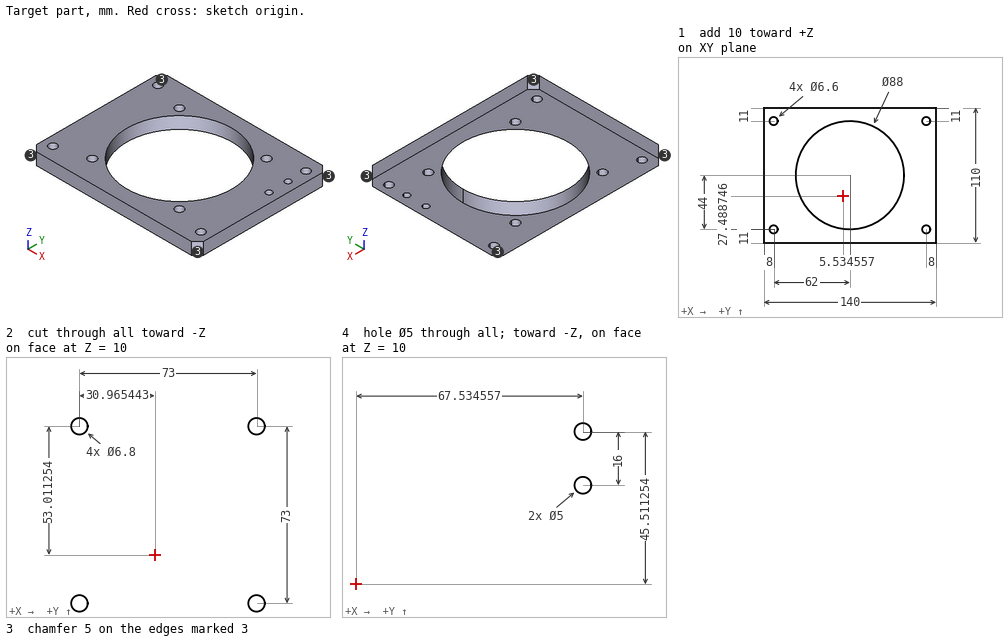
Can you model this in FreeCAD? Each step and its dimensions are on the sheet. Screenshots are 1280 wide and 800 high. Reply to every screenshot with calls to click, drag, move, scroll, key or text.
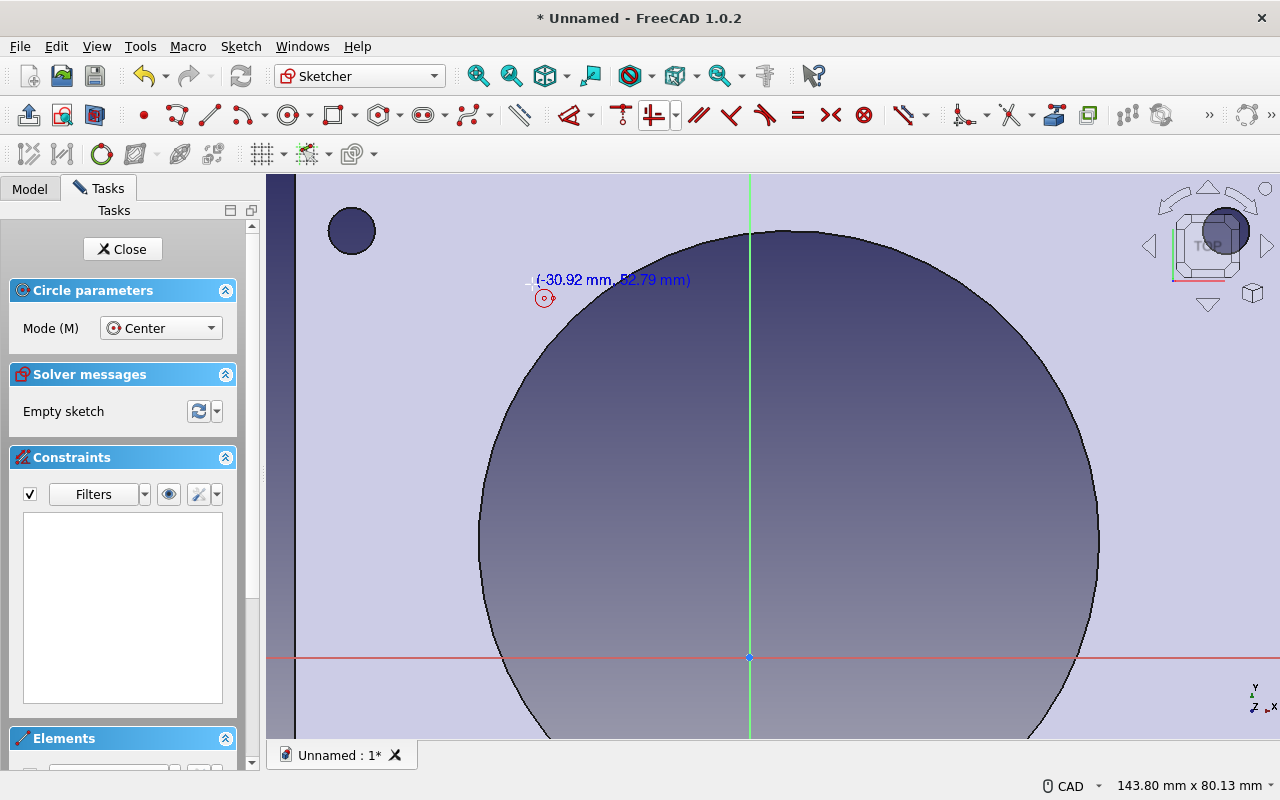
click(532, 284)
move(549, 267)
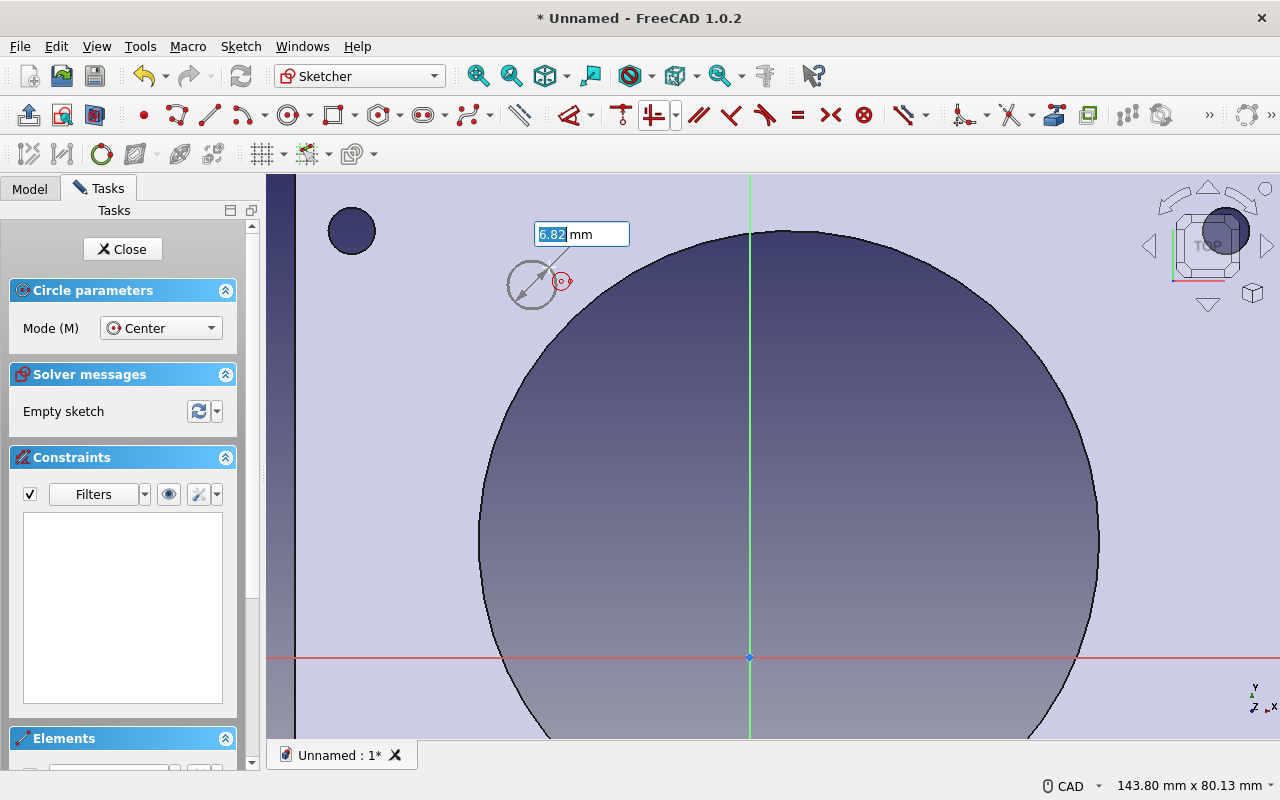
text(6.8)
key(Return)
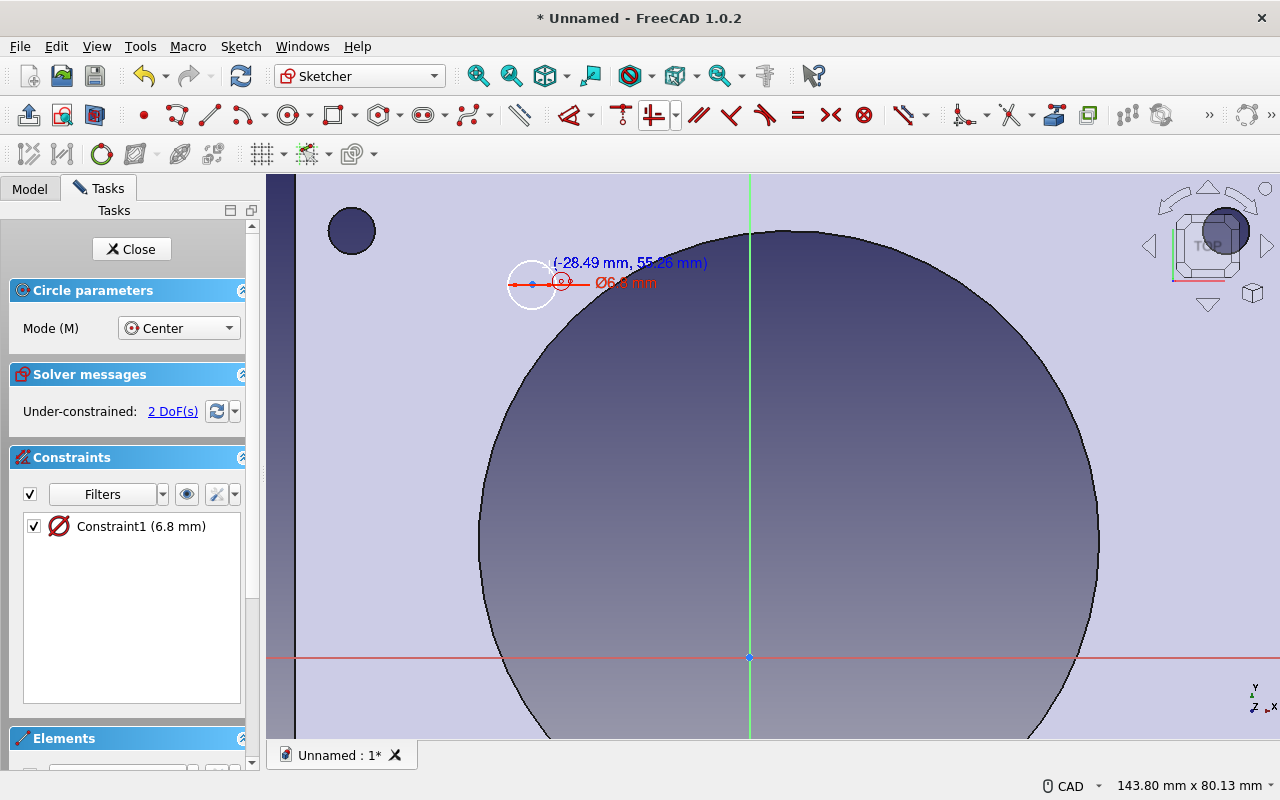
click(1046, 284)
move(1063, 267)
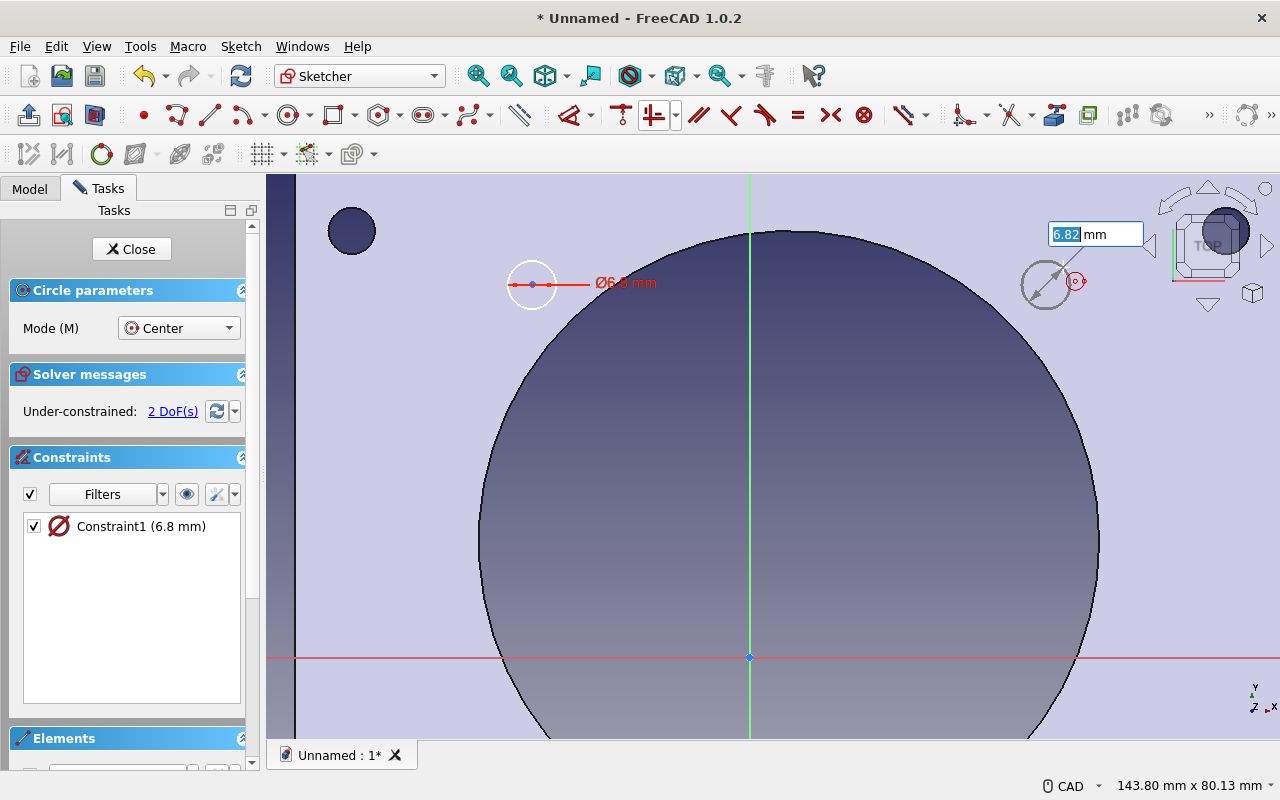
text(6.8)
key(Return)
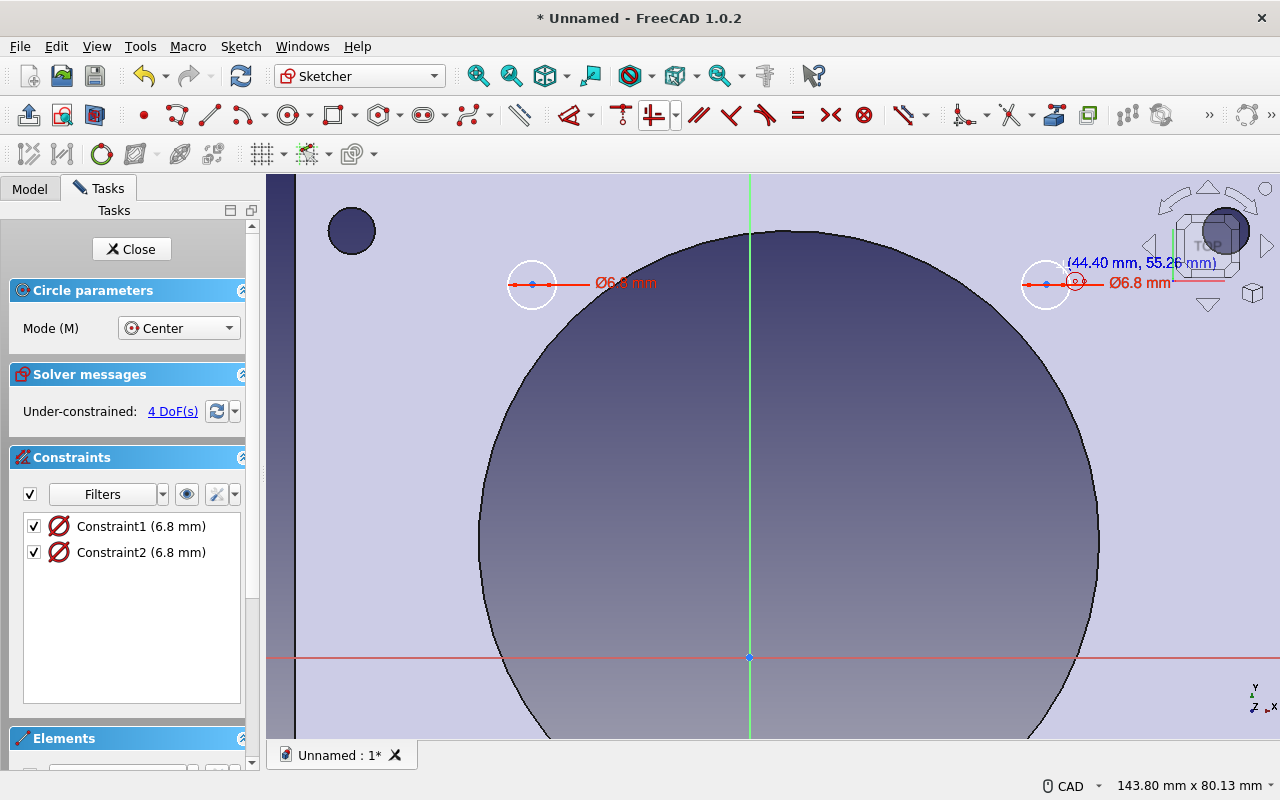
scroll(533, 284, down, 2)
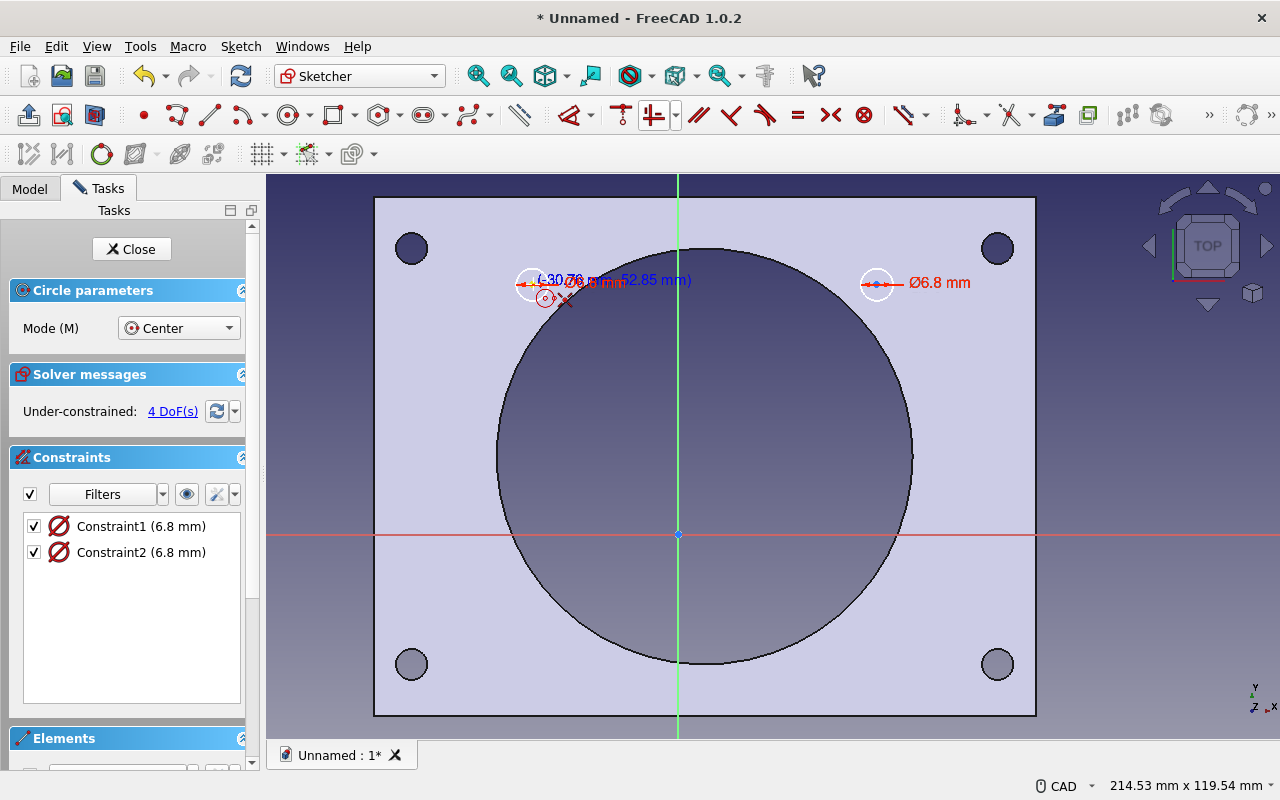
scroll(877, 629, up, 2)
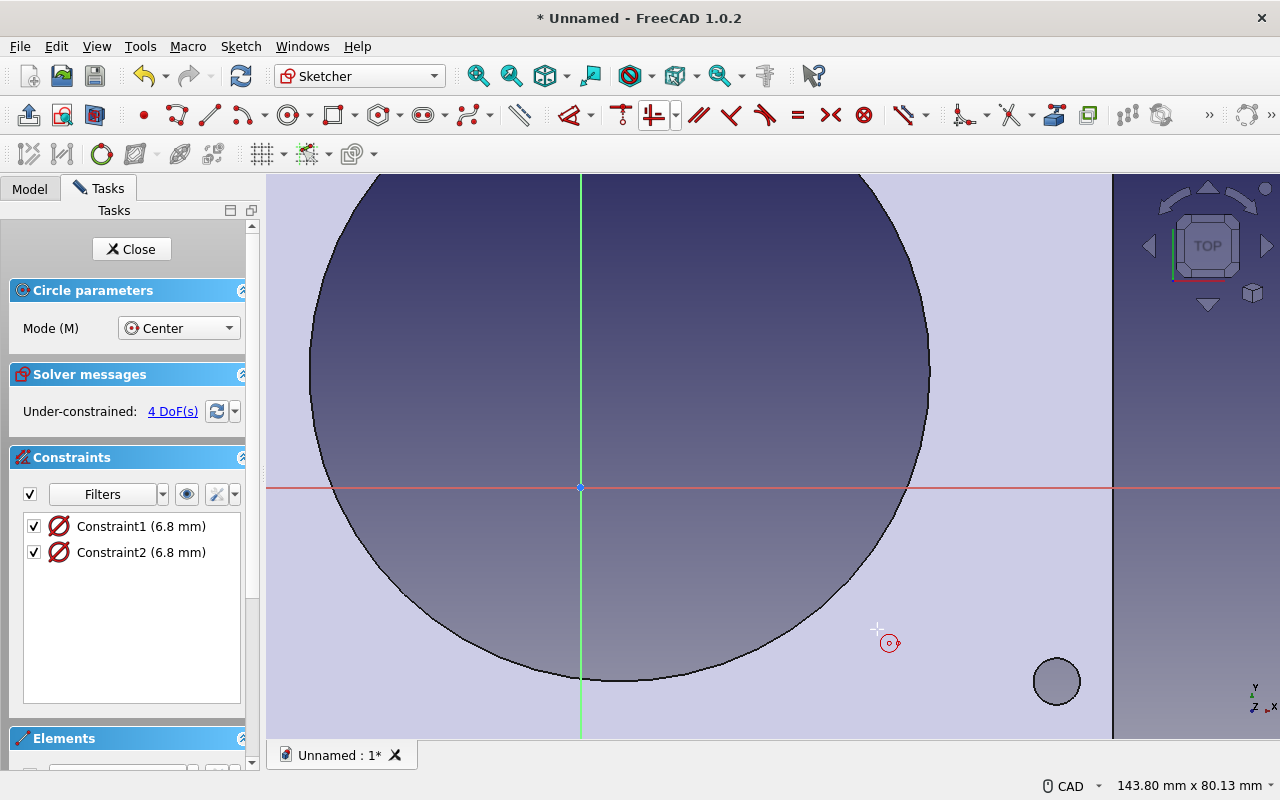
click(877, 629)
move(894, 612)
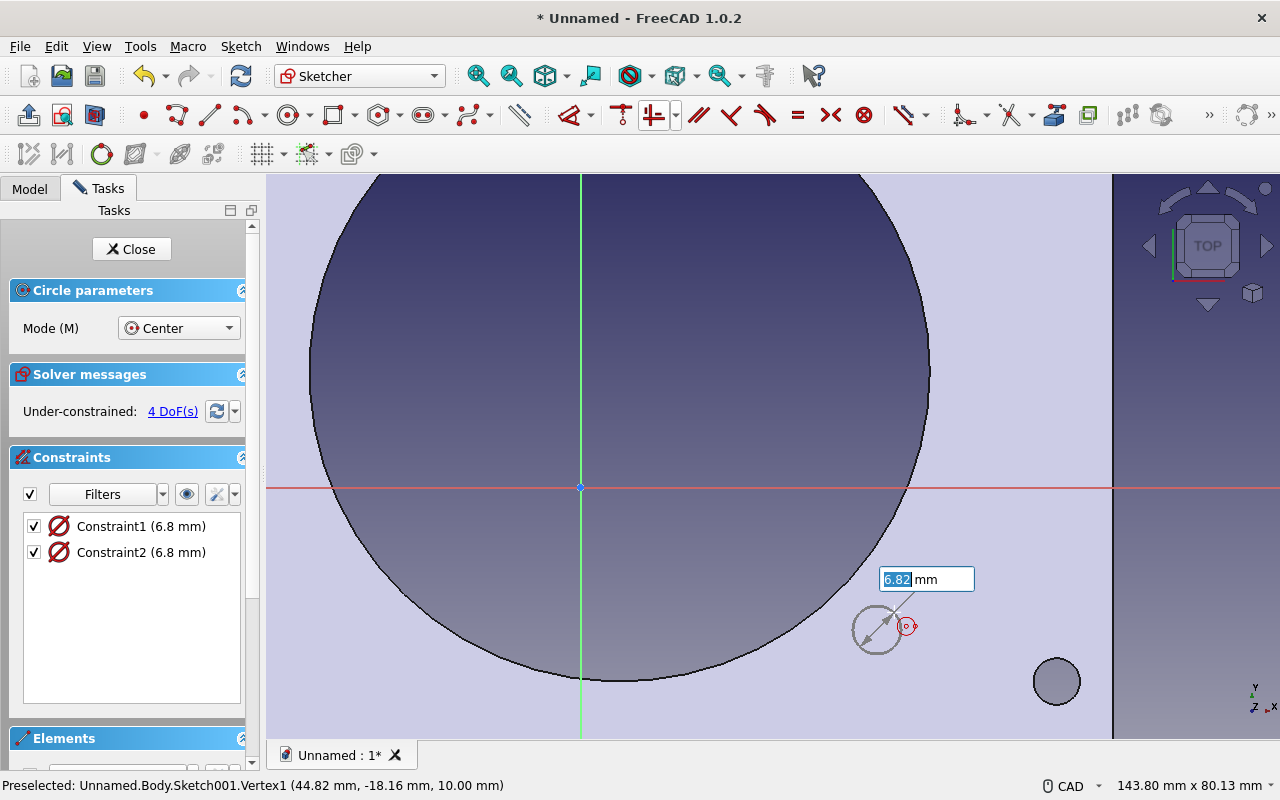
text(6.8)
key(Return)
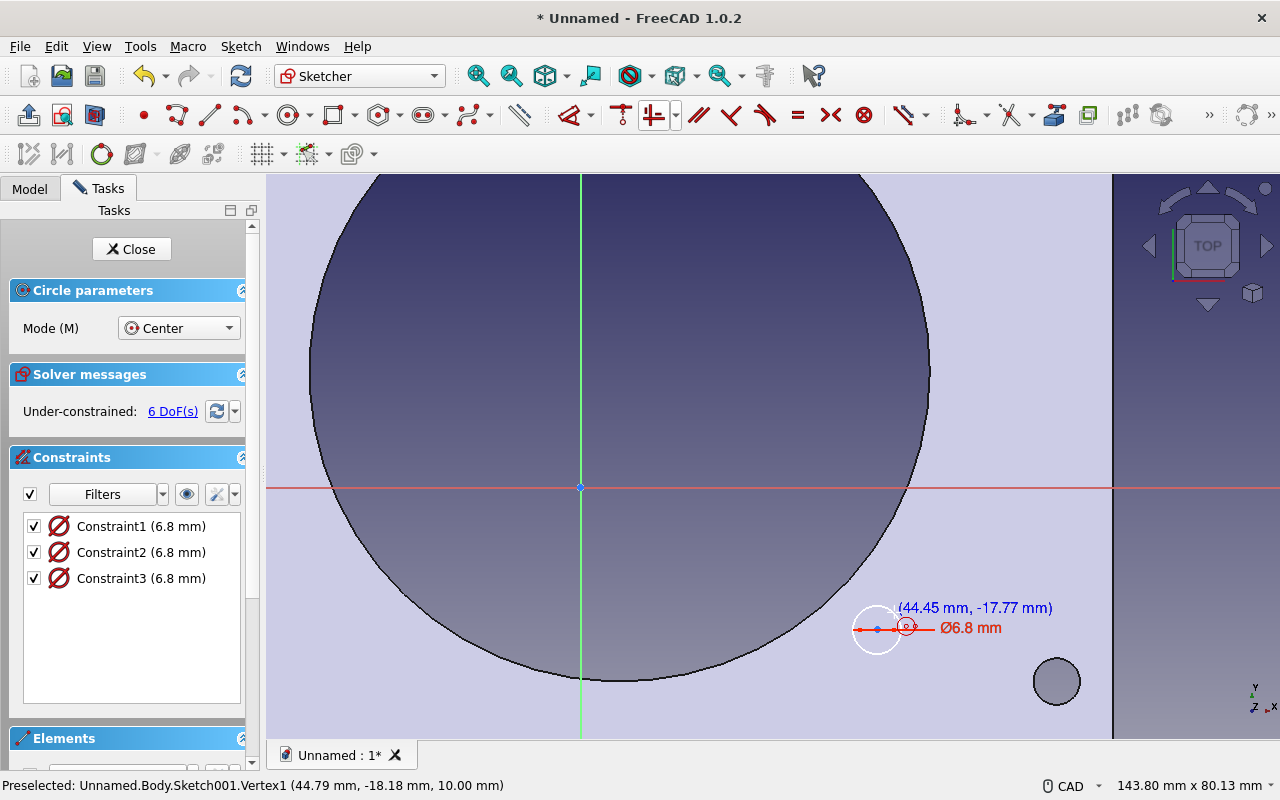
click(362, 629)
move(379, 612)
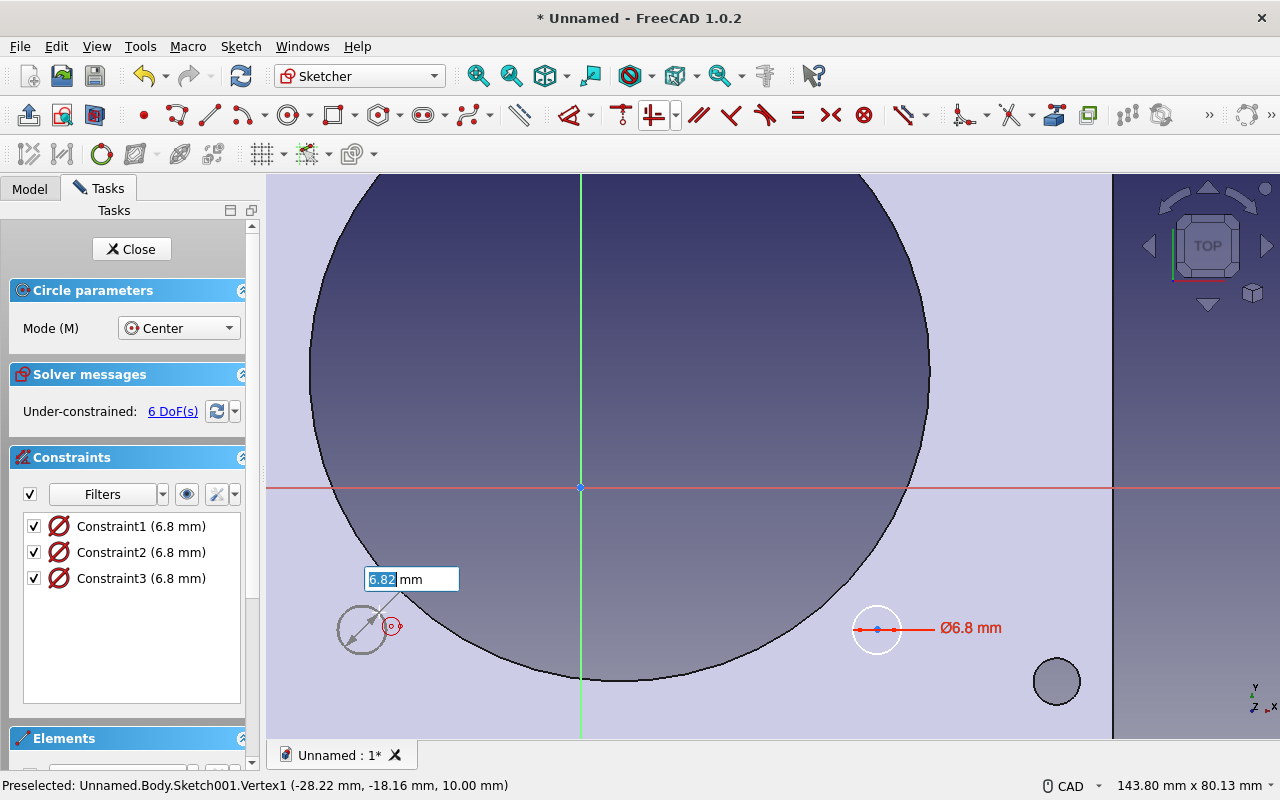
text(6.8)
key(Return)
key(Escape)